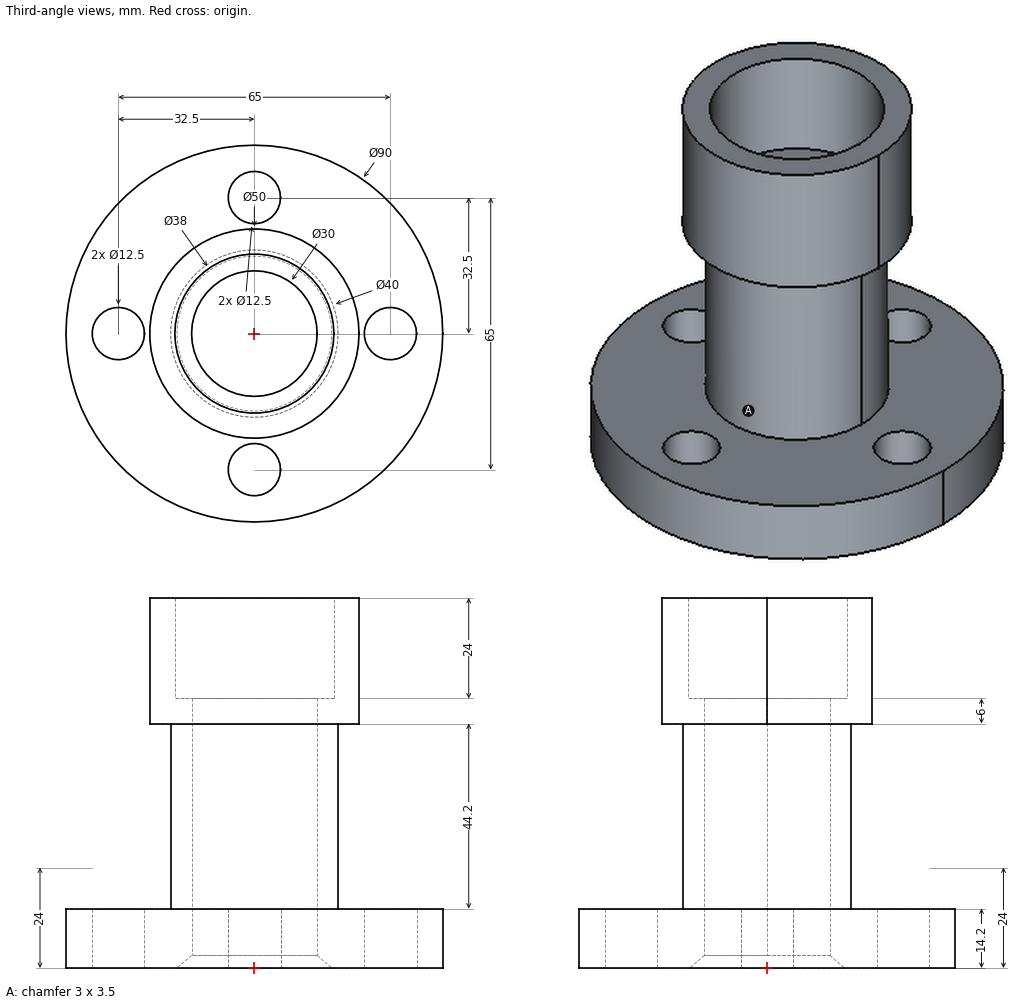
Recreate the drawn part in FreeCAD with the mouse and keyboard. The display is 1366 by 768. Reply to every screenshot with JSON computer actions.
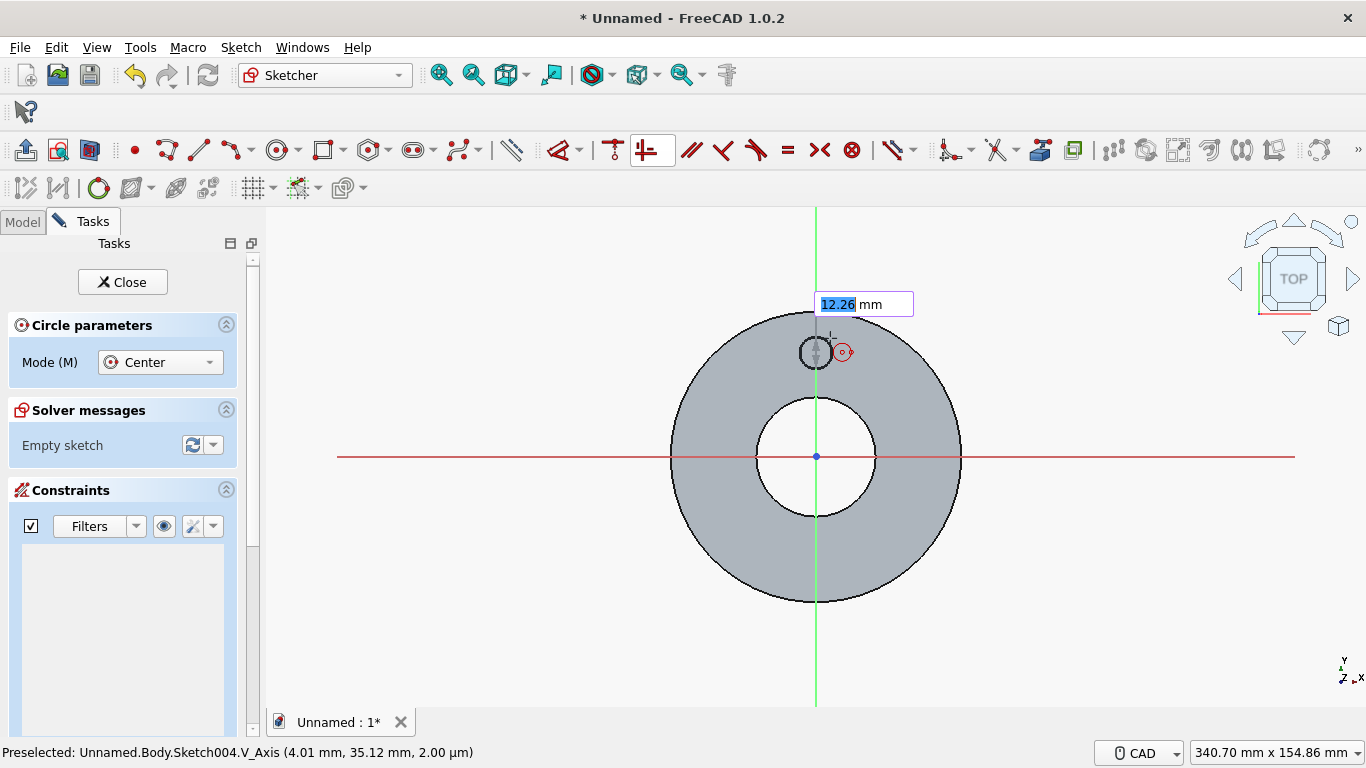
{"action": "type", "text": "12.5"}
{"action": "key", "text": "Return"}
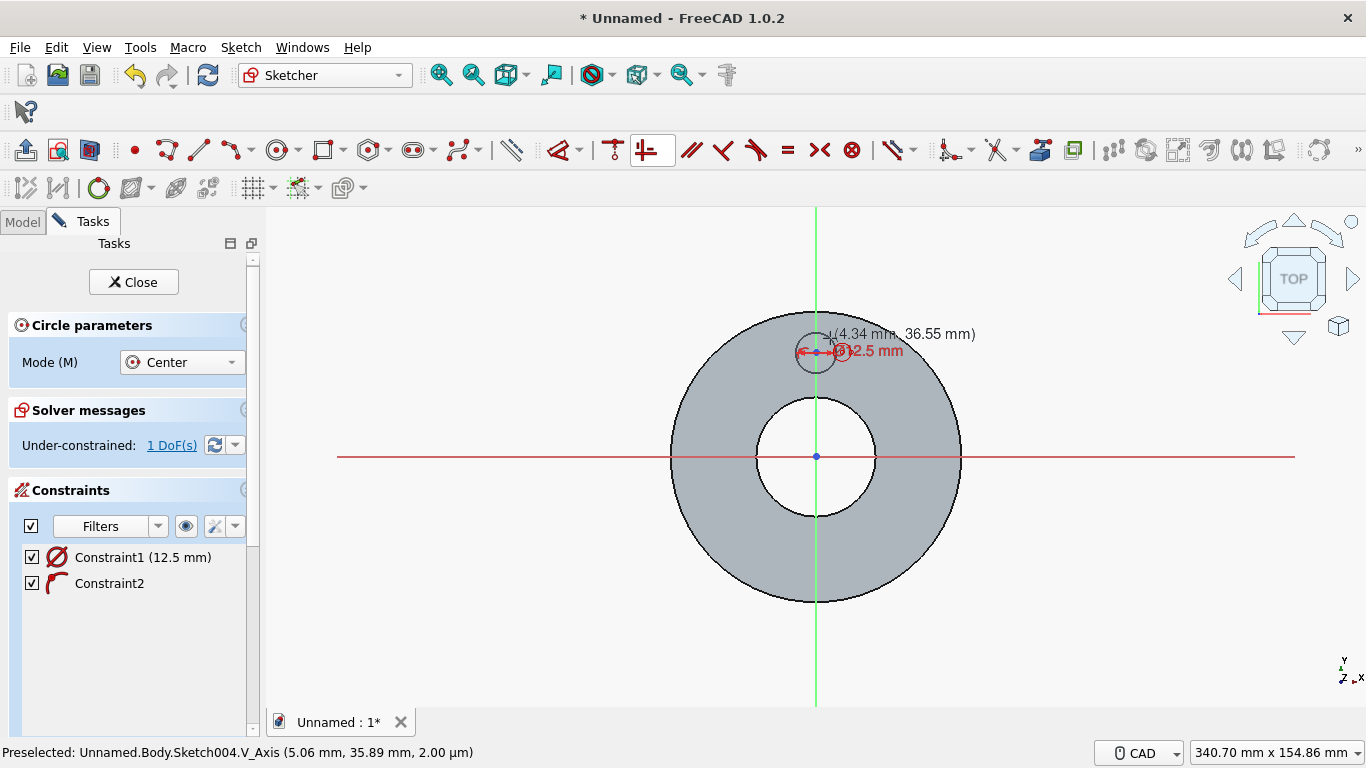
{"action": "left_click", "coordinate": [816, 562]}
{"action": "mouse_move", "coordinate": [830, 548]}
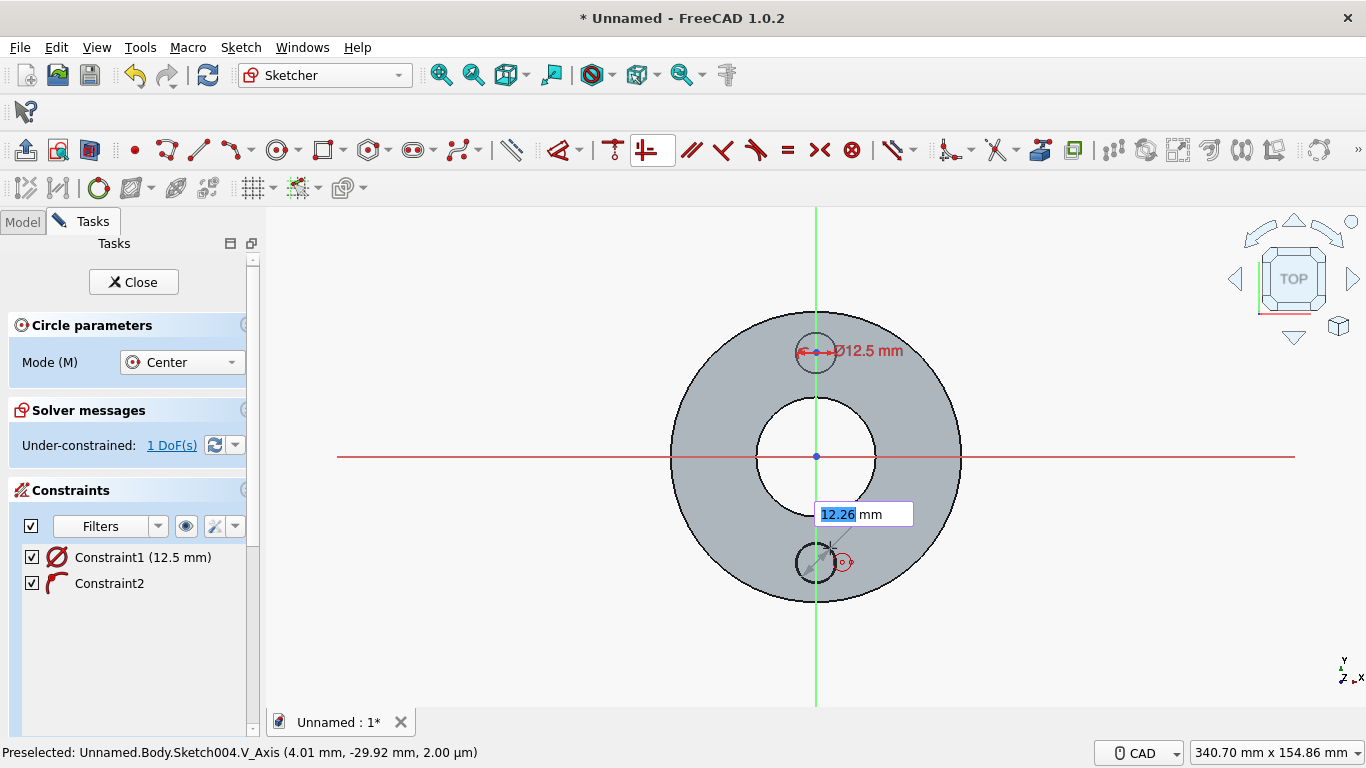
{"action": "type", "text": "12.5"}
{"action": "key", "text": "Return"}
{"action": "key", "text": "Escape"}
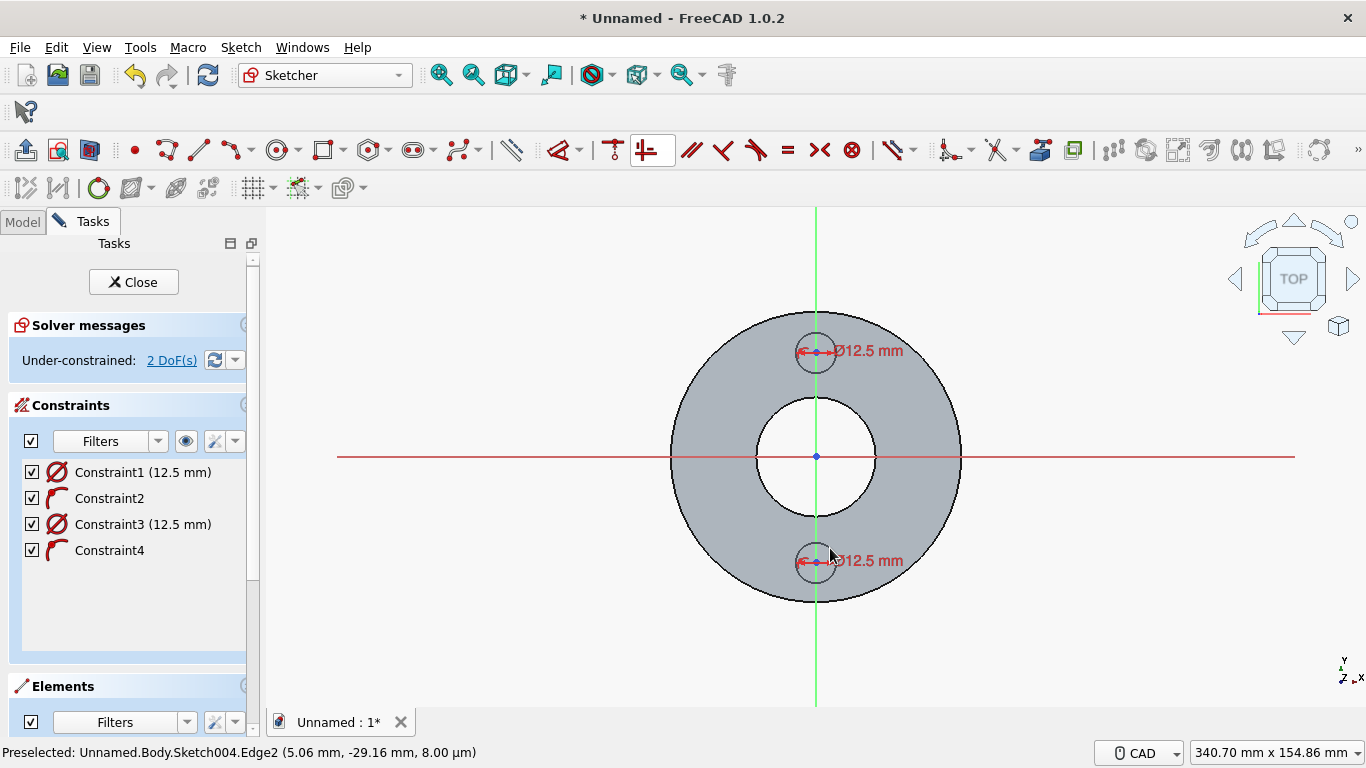
{"action": "left_click", "coordinate": [816, 353]}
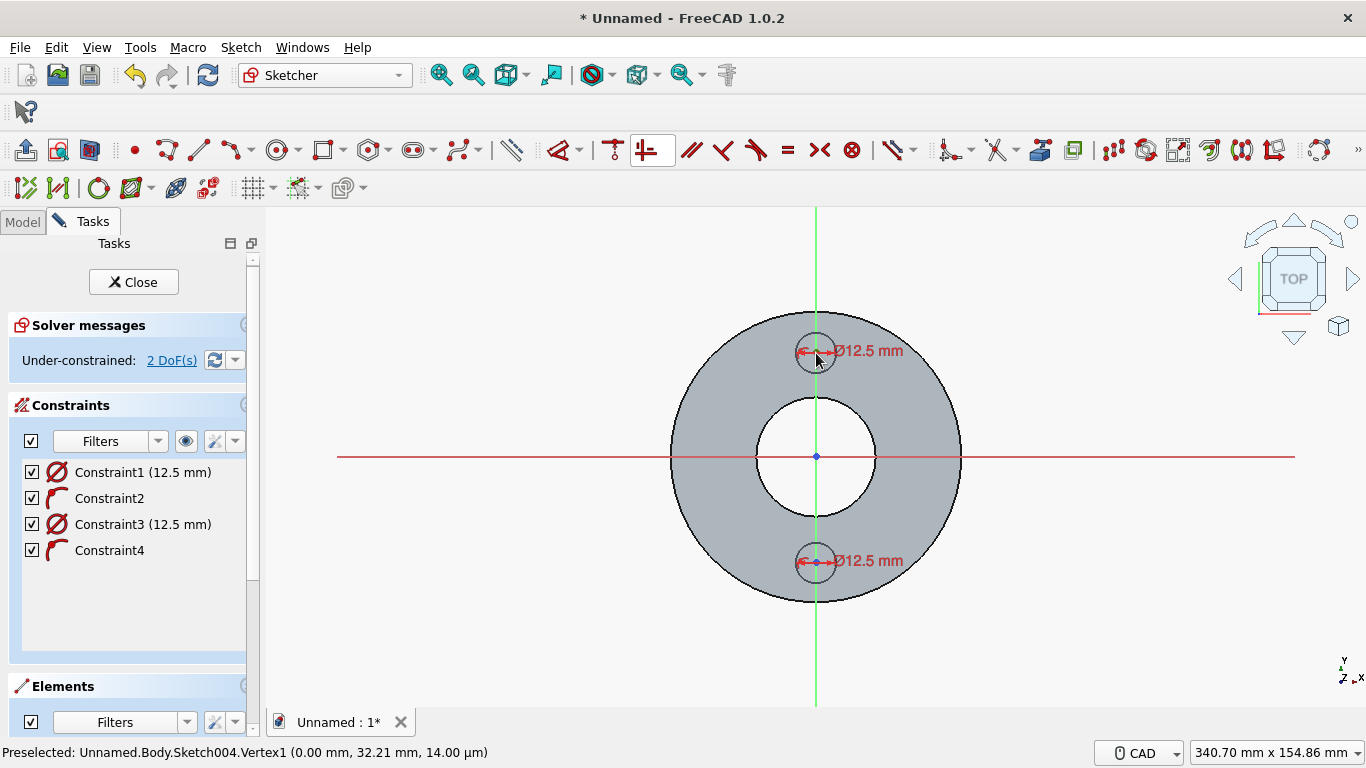
{"action": "left_click", "coordinate": [816, 563]}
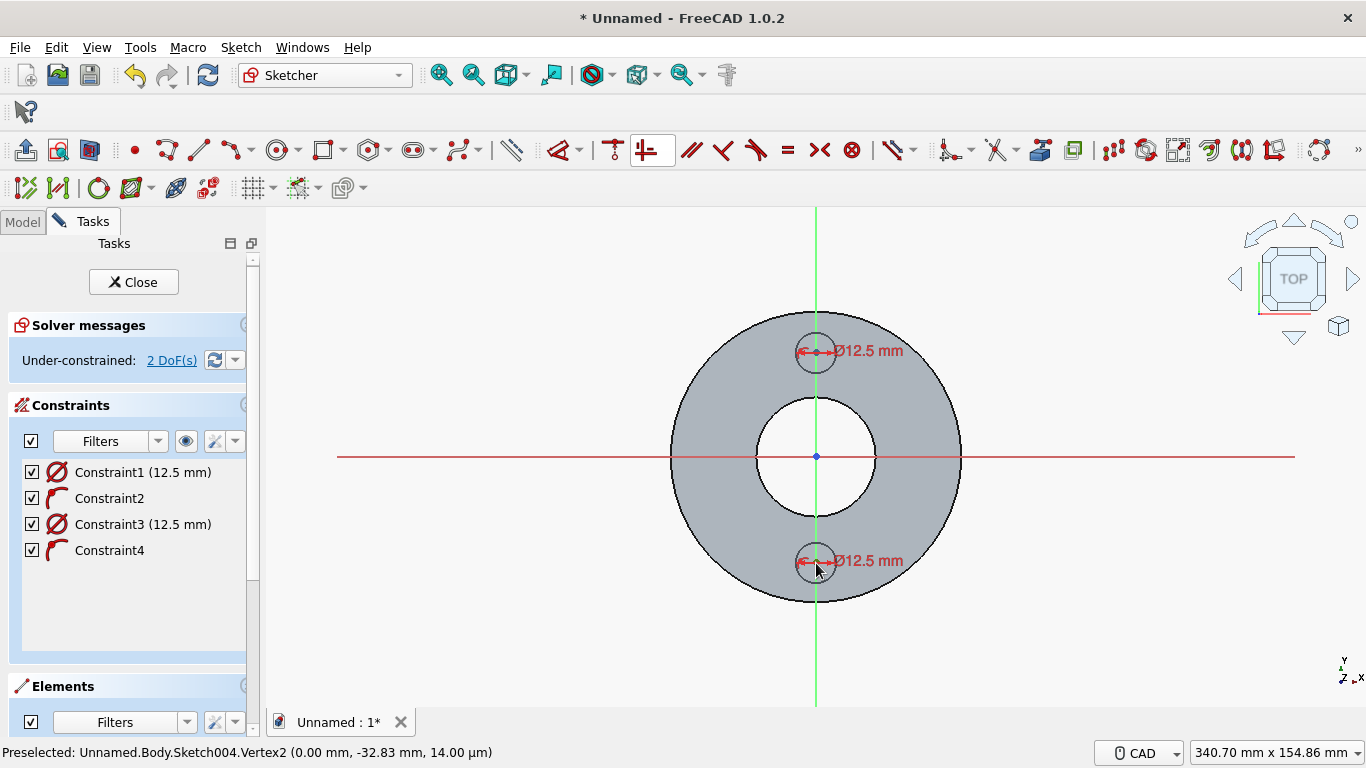
{"action": "left_click", "coordinate": [582, 150]}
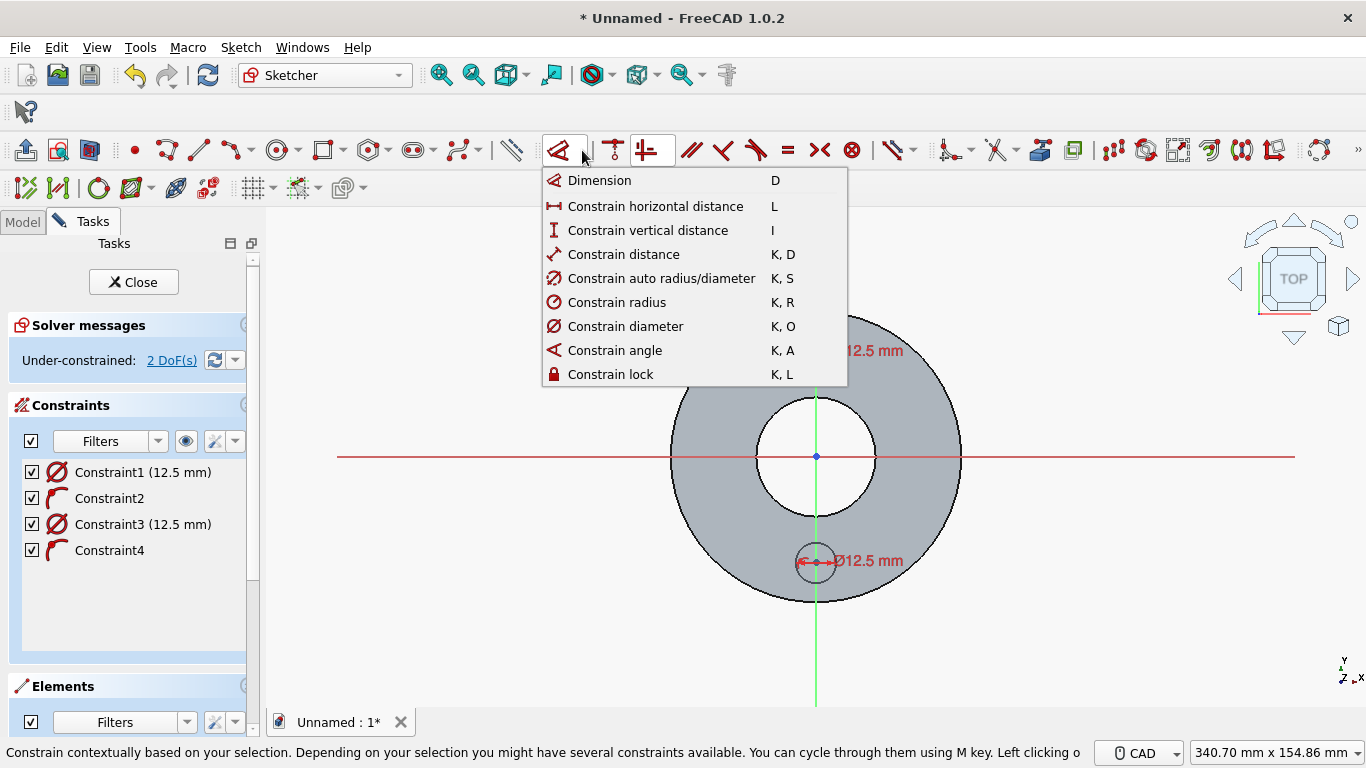
{"action": "left_click", "coordinate": [695, 230]}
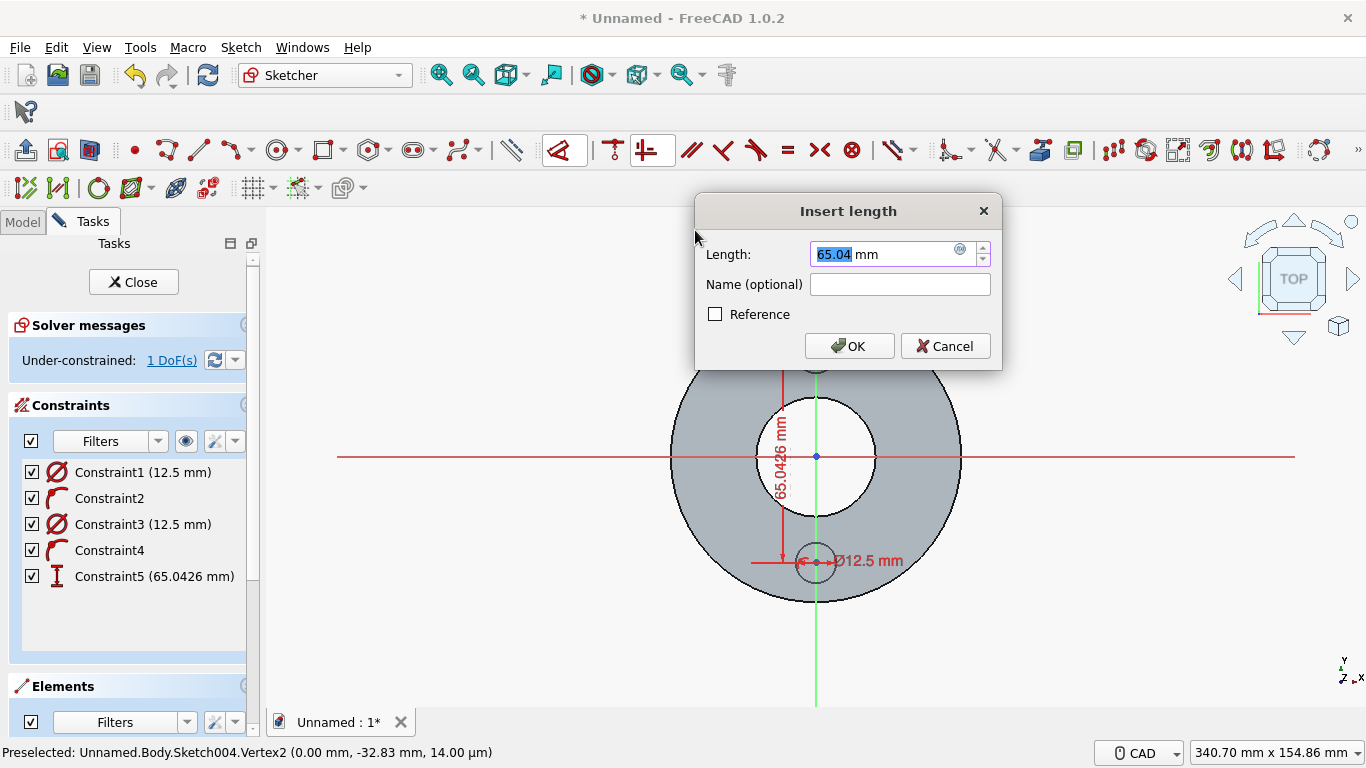
{"action": "type", "text": "65"}
{"action": "key", "text": "Return"}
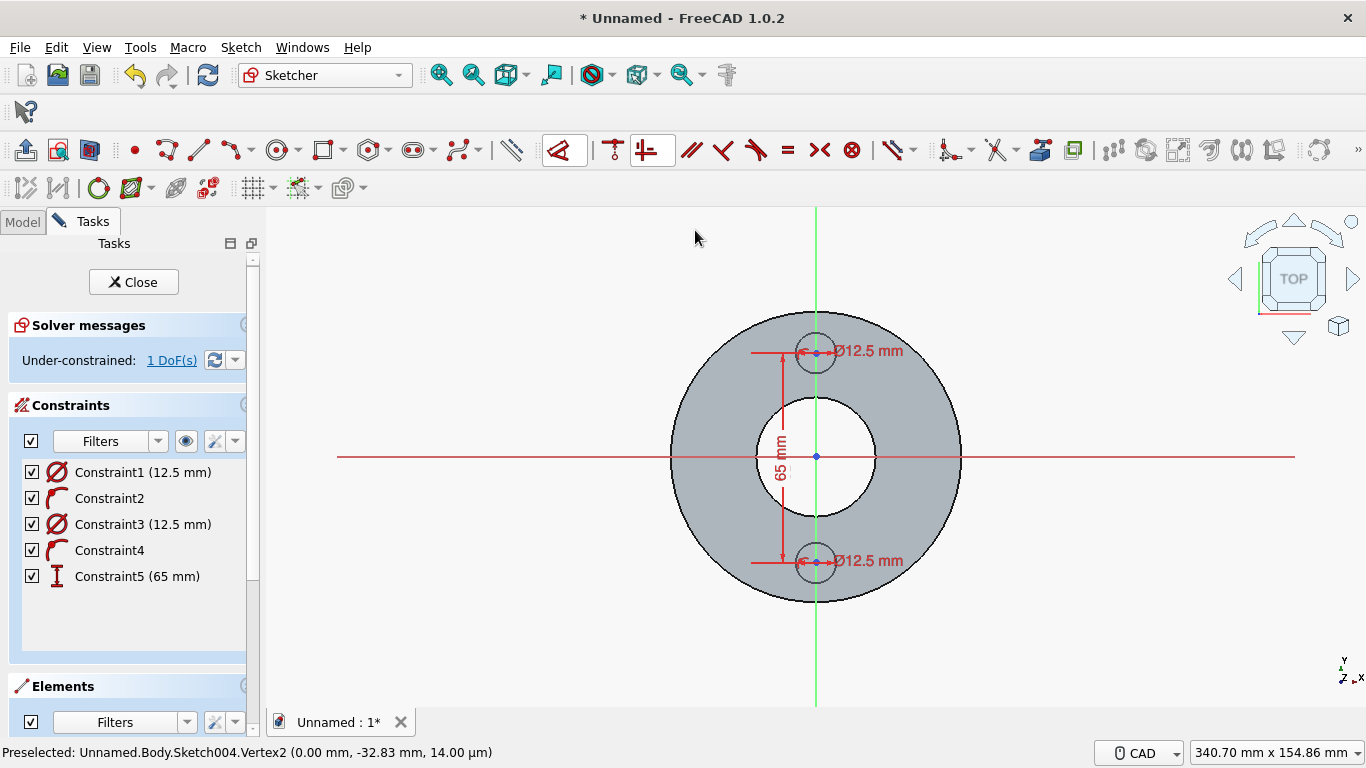
{"action": "left_click", "coordinate": [816, 353]}